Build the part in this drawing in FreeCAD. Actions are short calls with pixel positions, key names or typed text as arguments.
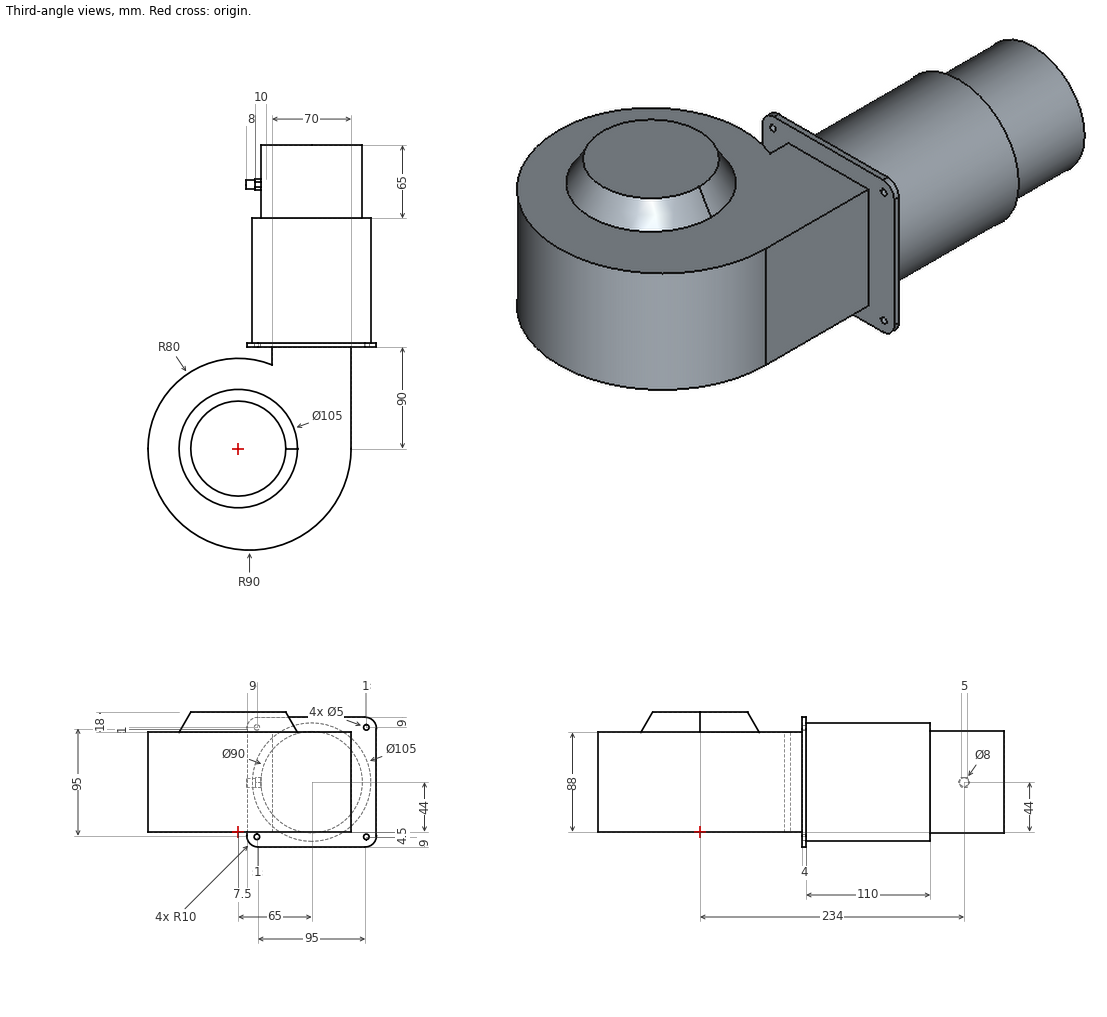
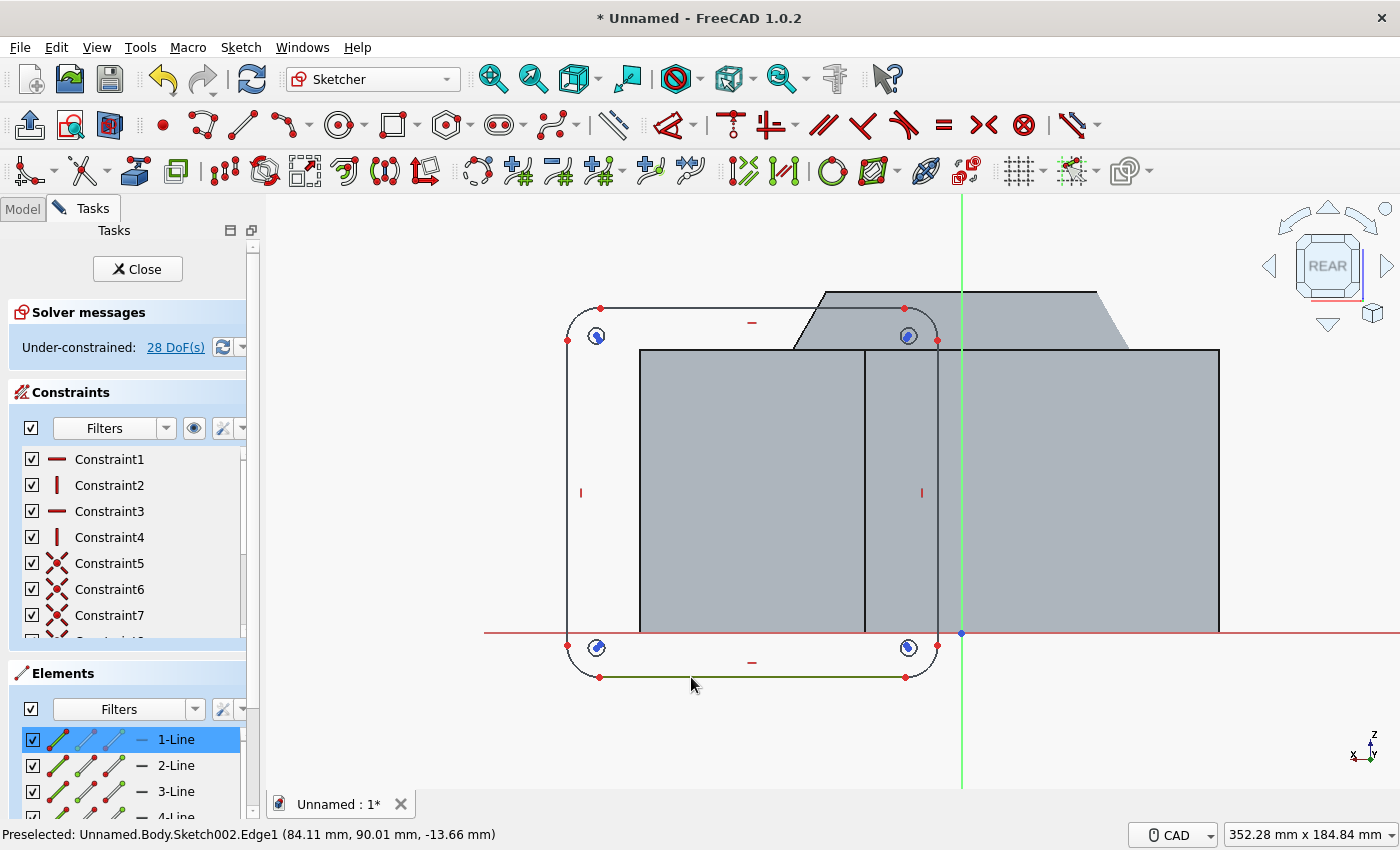
click(920, 674)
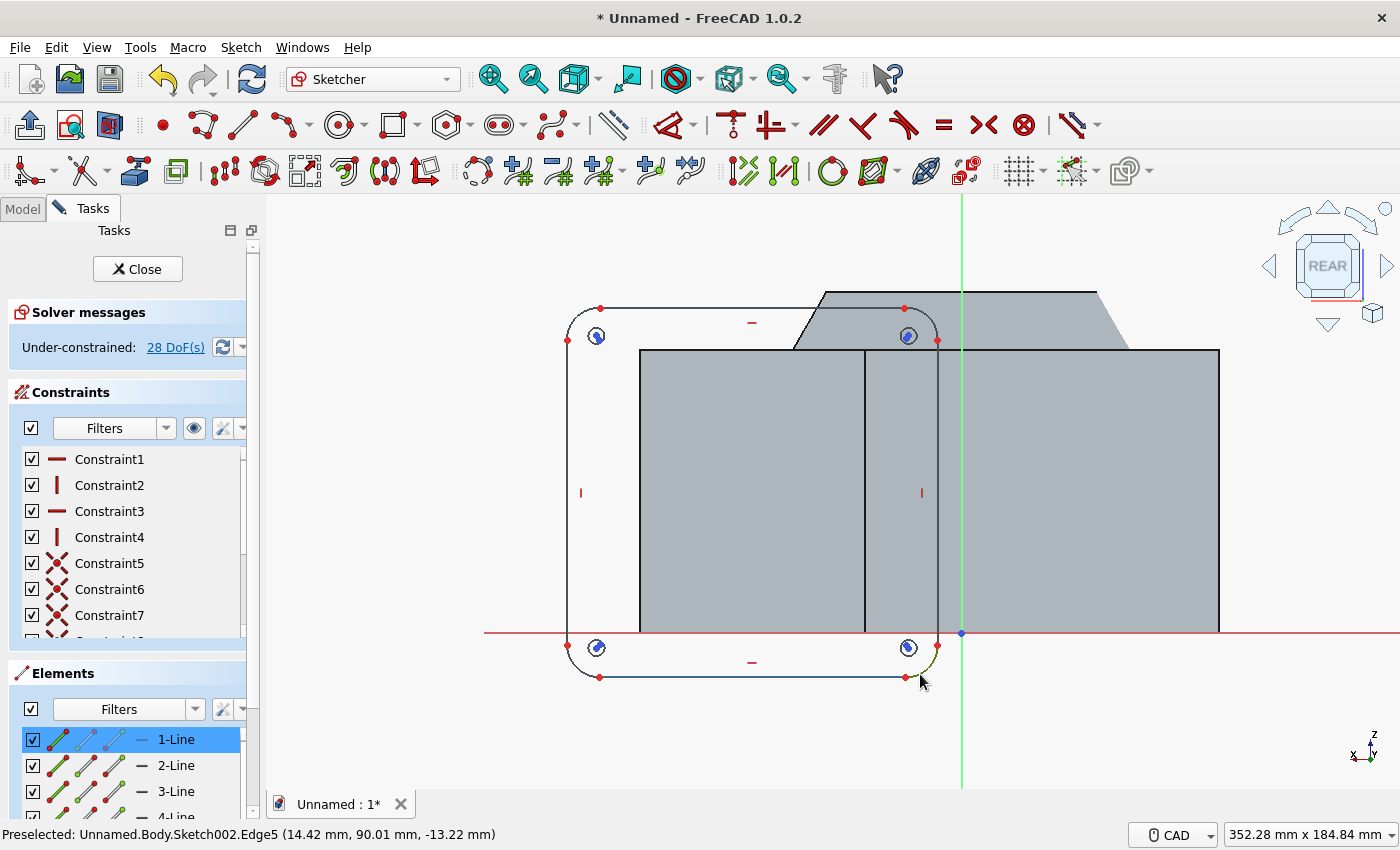
click(904, 126)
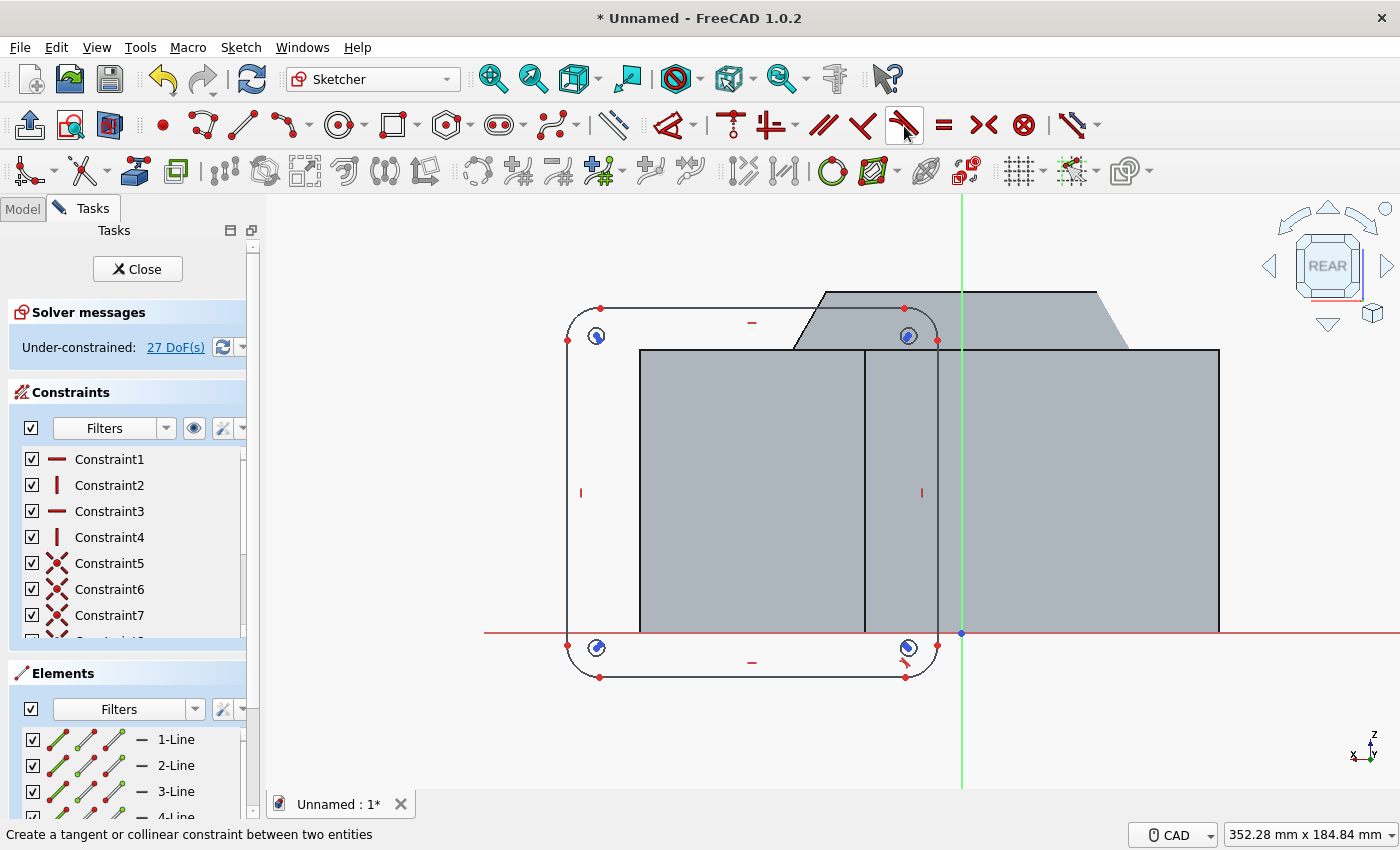
click(691, 677)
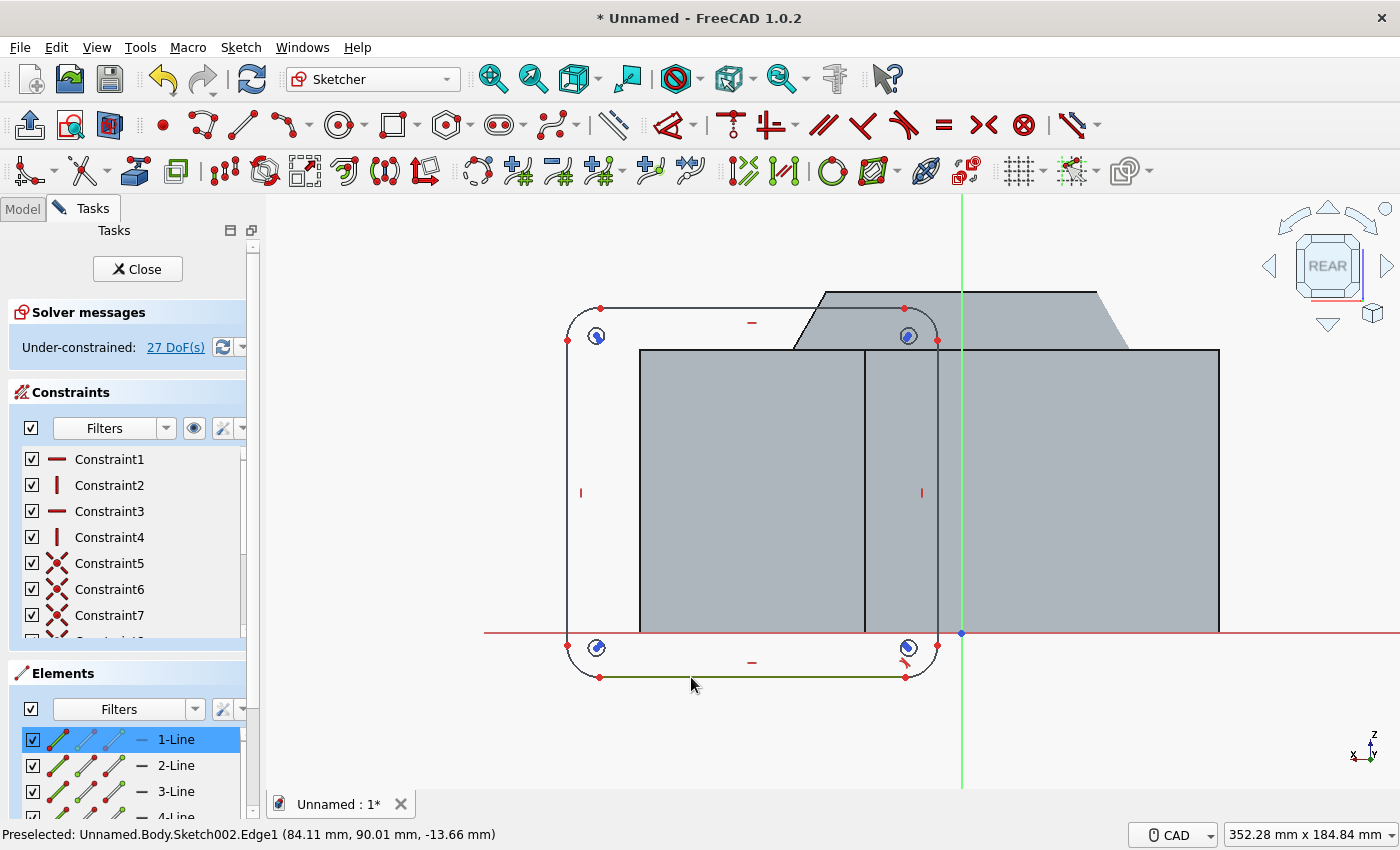
click(571, 660)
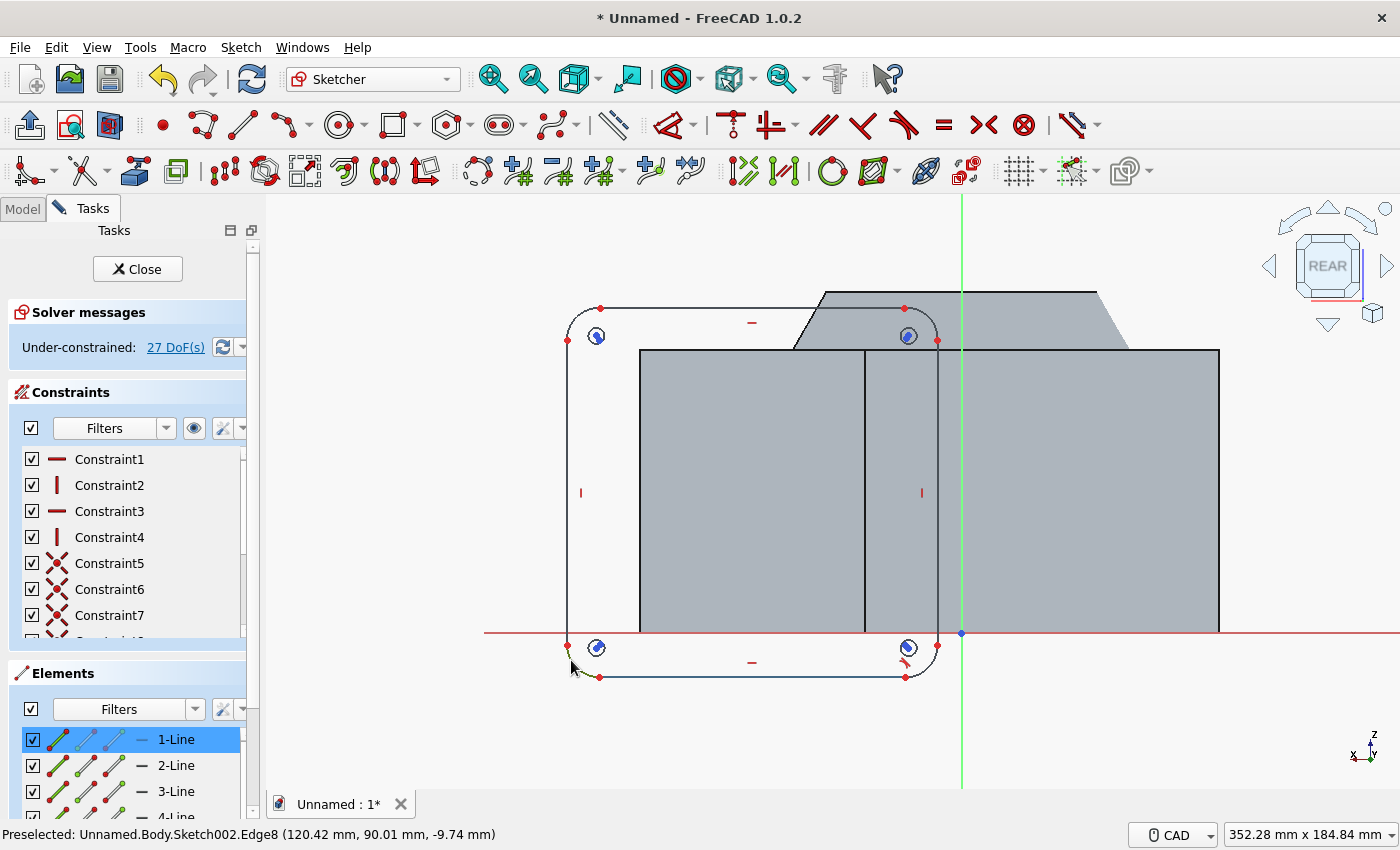
click(904, 126)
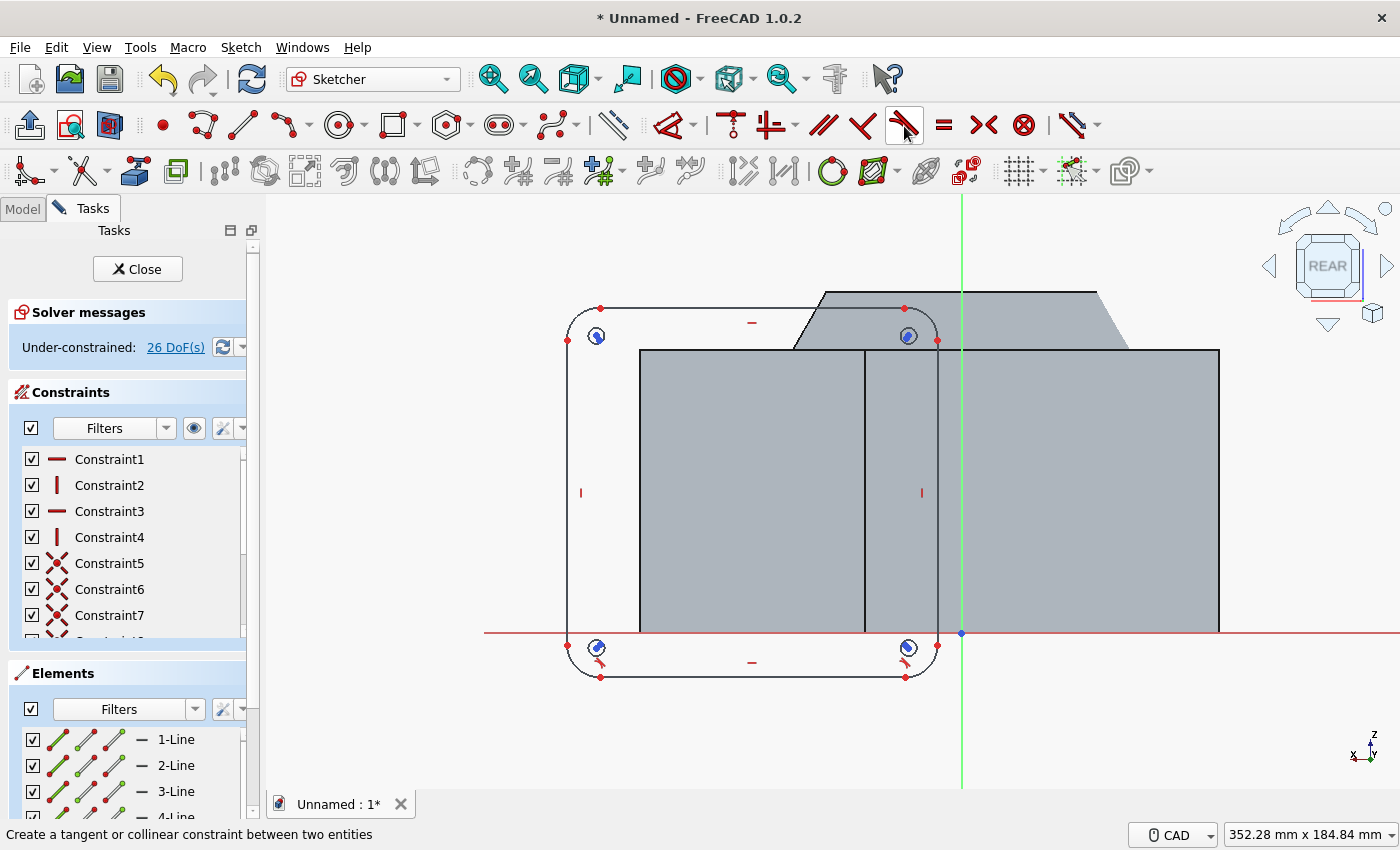
click(938, 554)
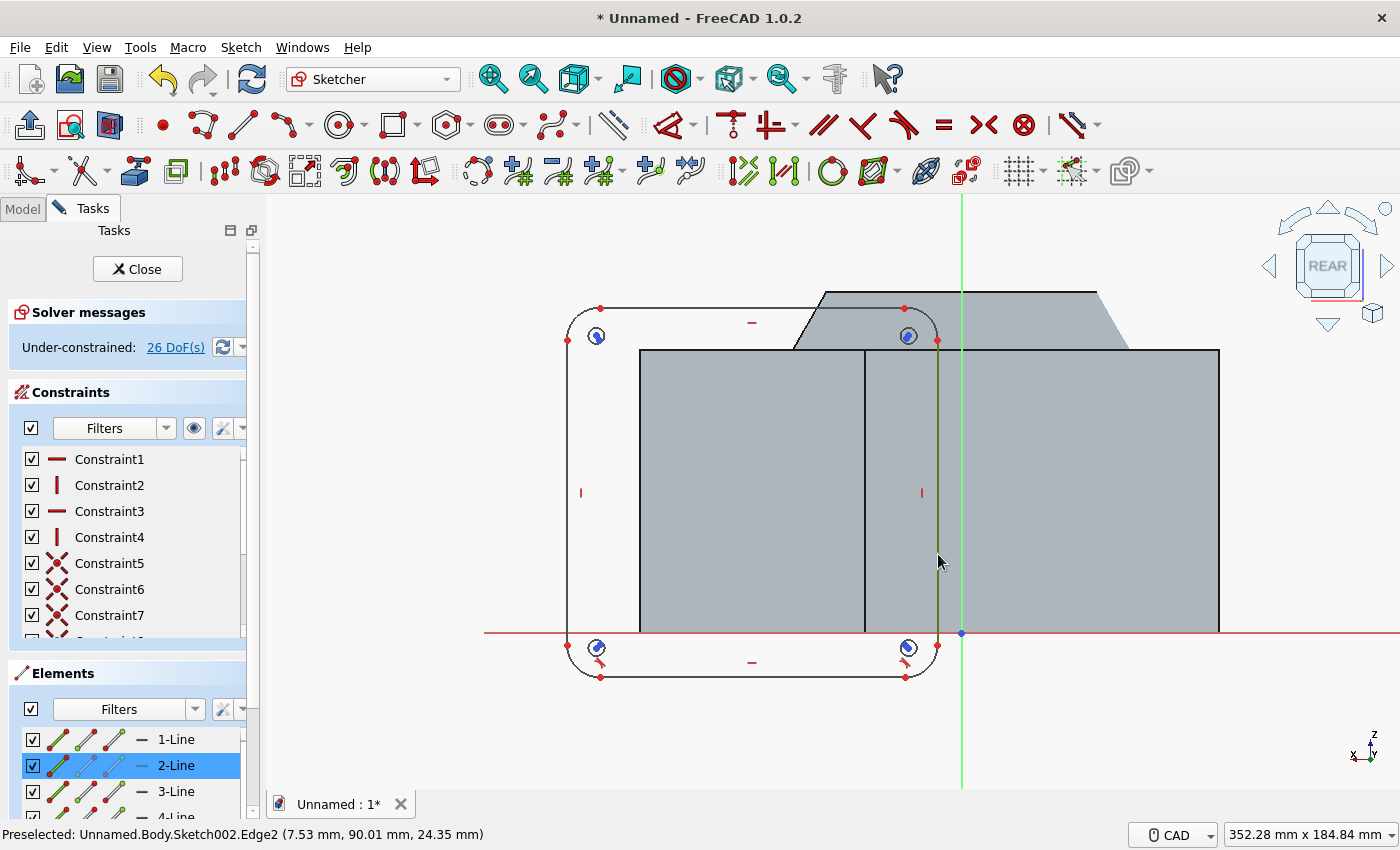
click(920, 674)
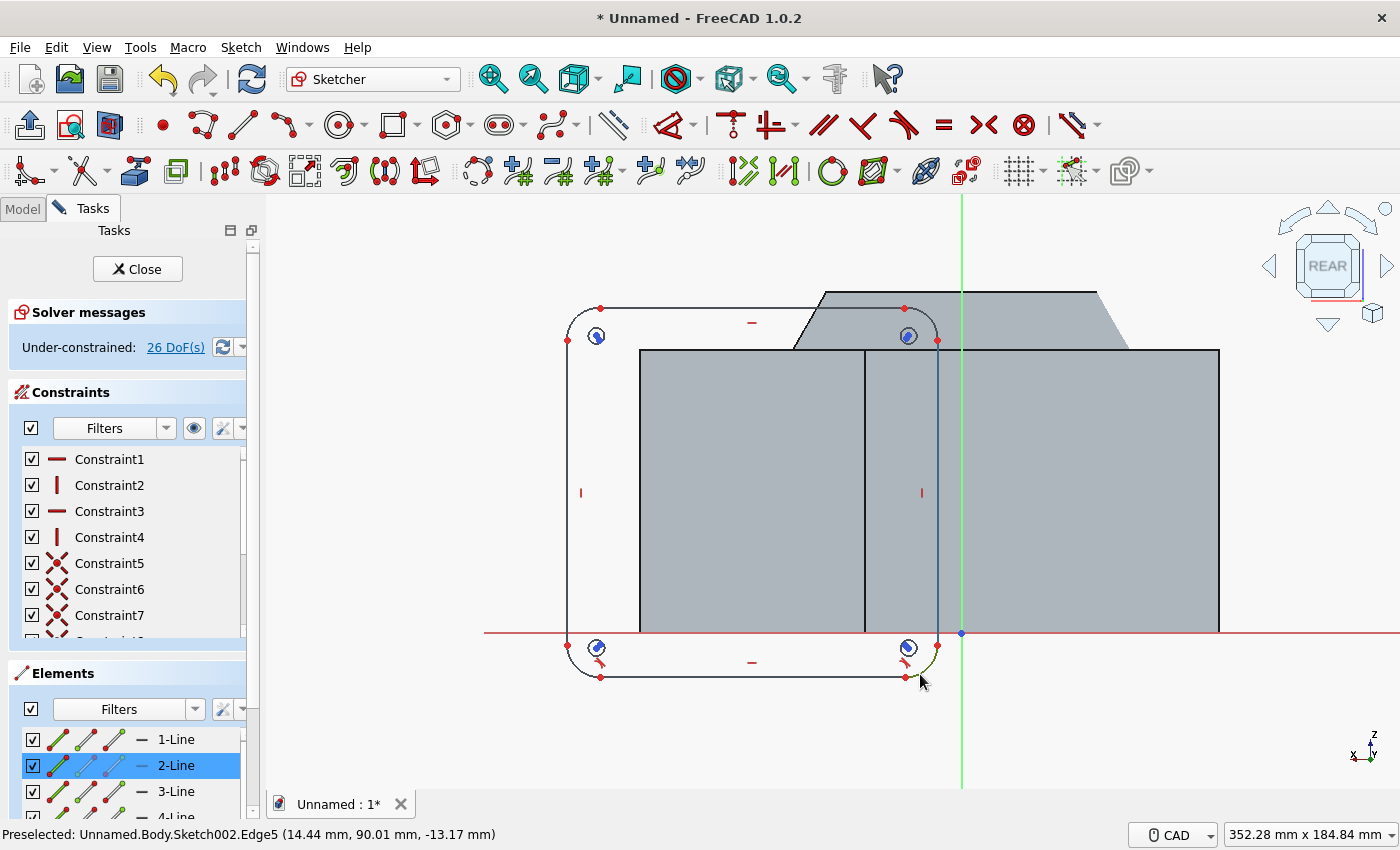
click(904, 126)